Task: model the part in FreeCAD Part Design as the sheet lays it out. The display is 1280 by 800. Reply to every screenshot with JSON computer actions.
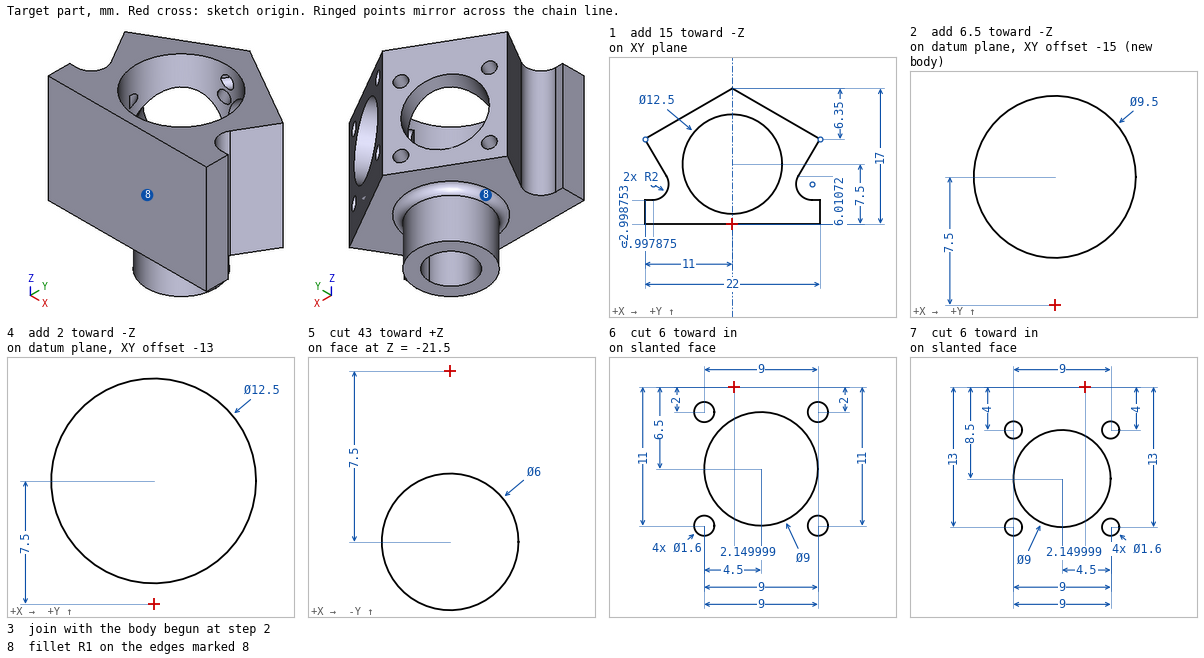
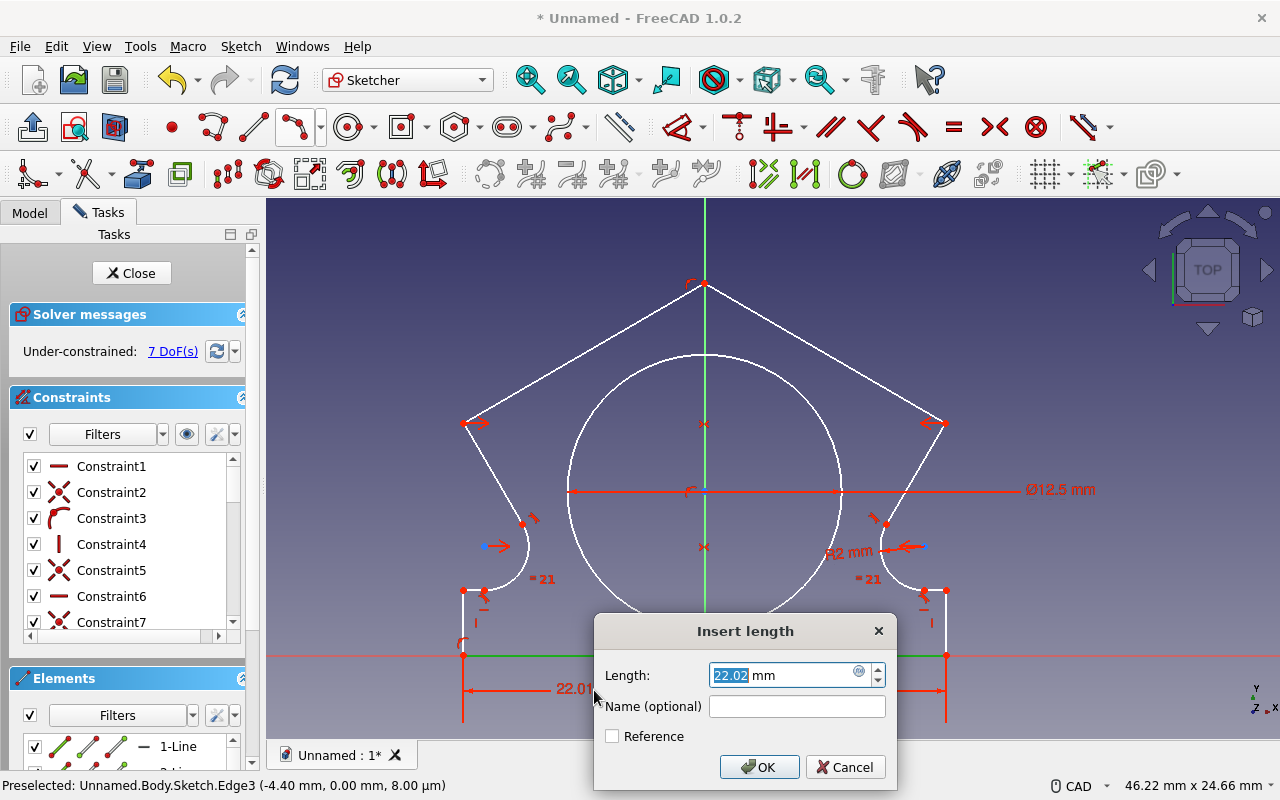
{"action": "type", "text": "22"}
{"action": "key", "text": "Return"}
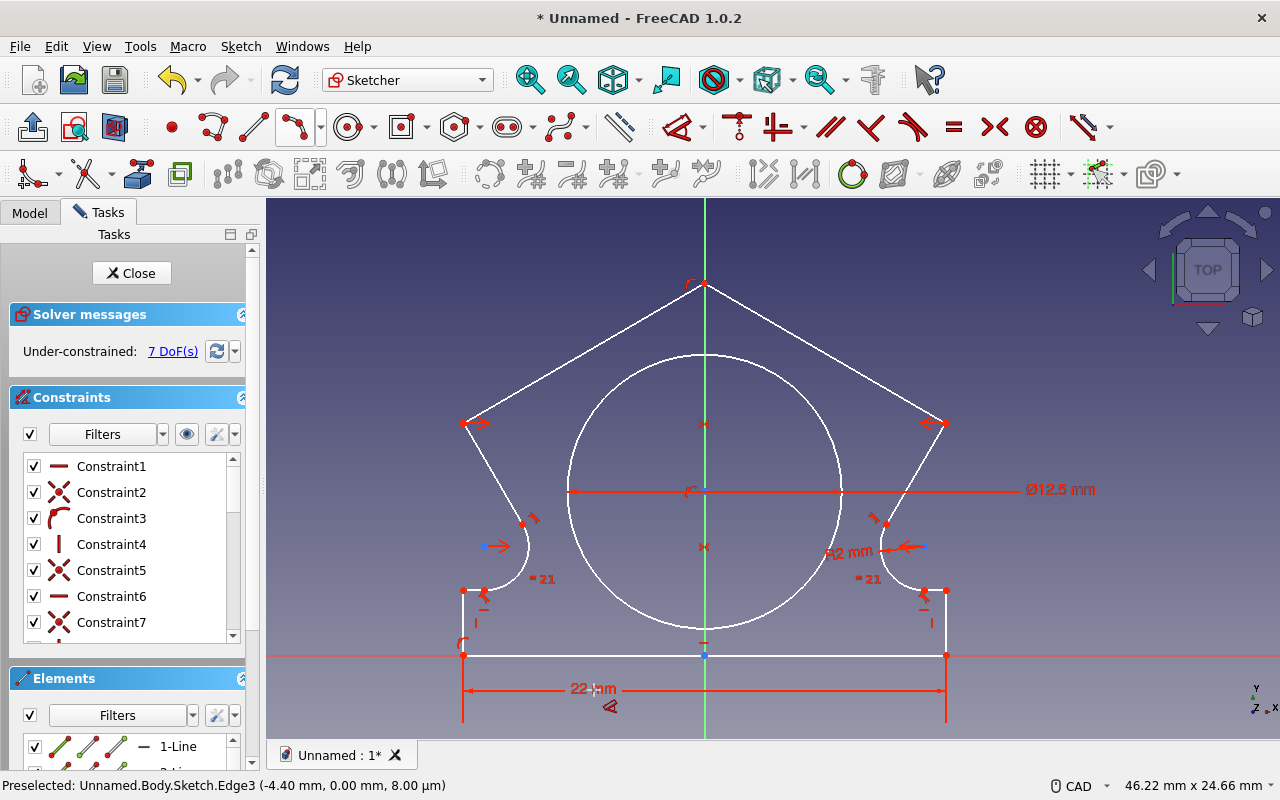
{"action": "left_click", "coordinate": [463, 590]}
{"action": "left_click", "coordinate": [500, 690]}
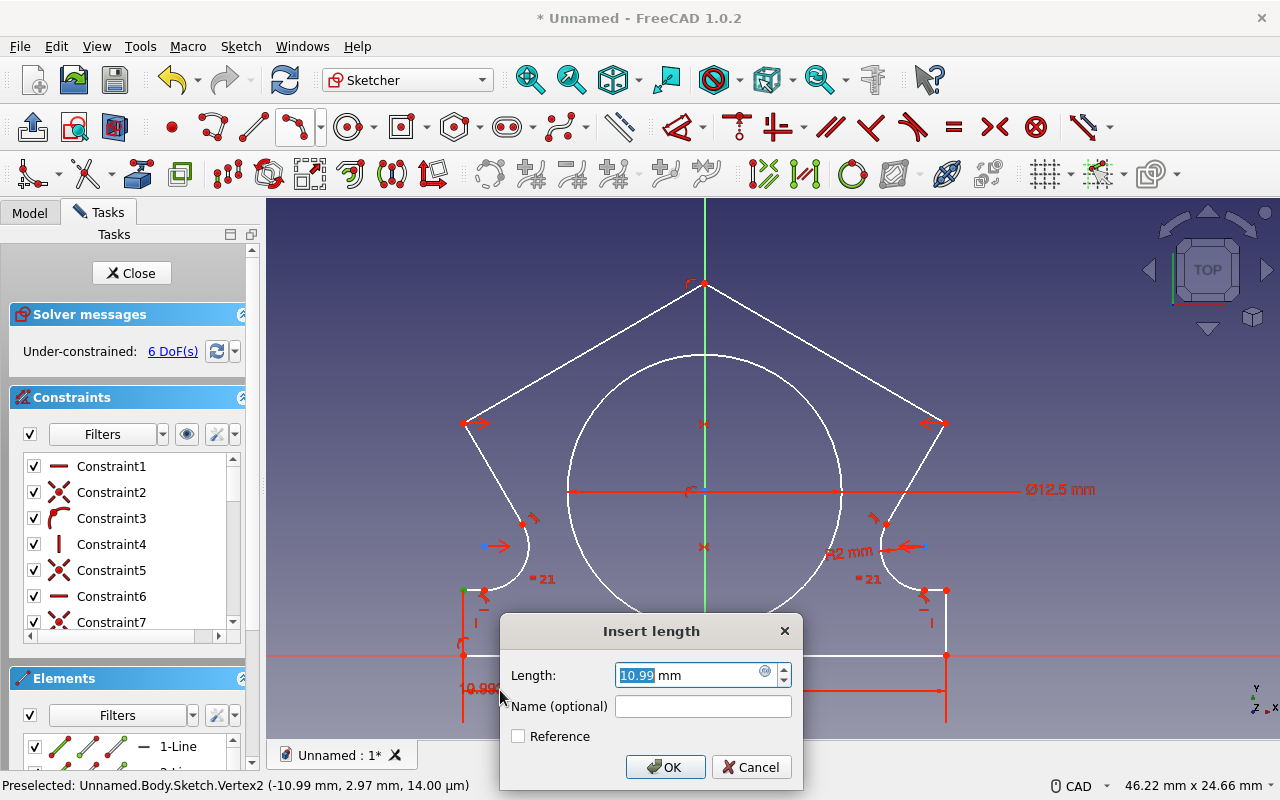
{"action": "type", "text": "11"}
{"action": "key", "text": "Return"}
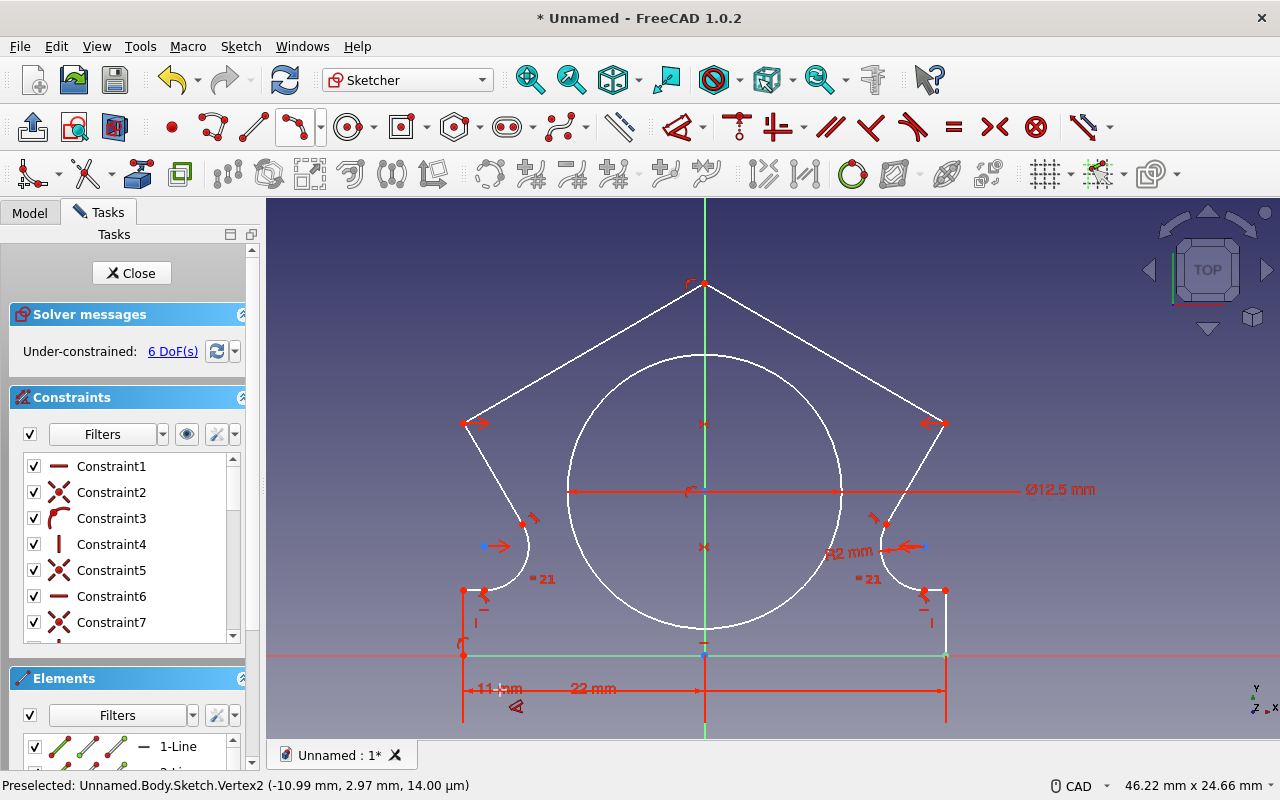
{"action": "left_click", "coordinate": [705, 283]}
{"action": "left_click", "coordinate": [739, 469]}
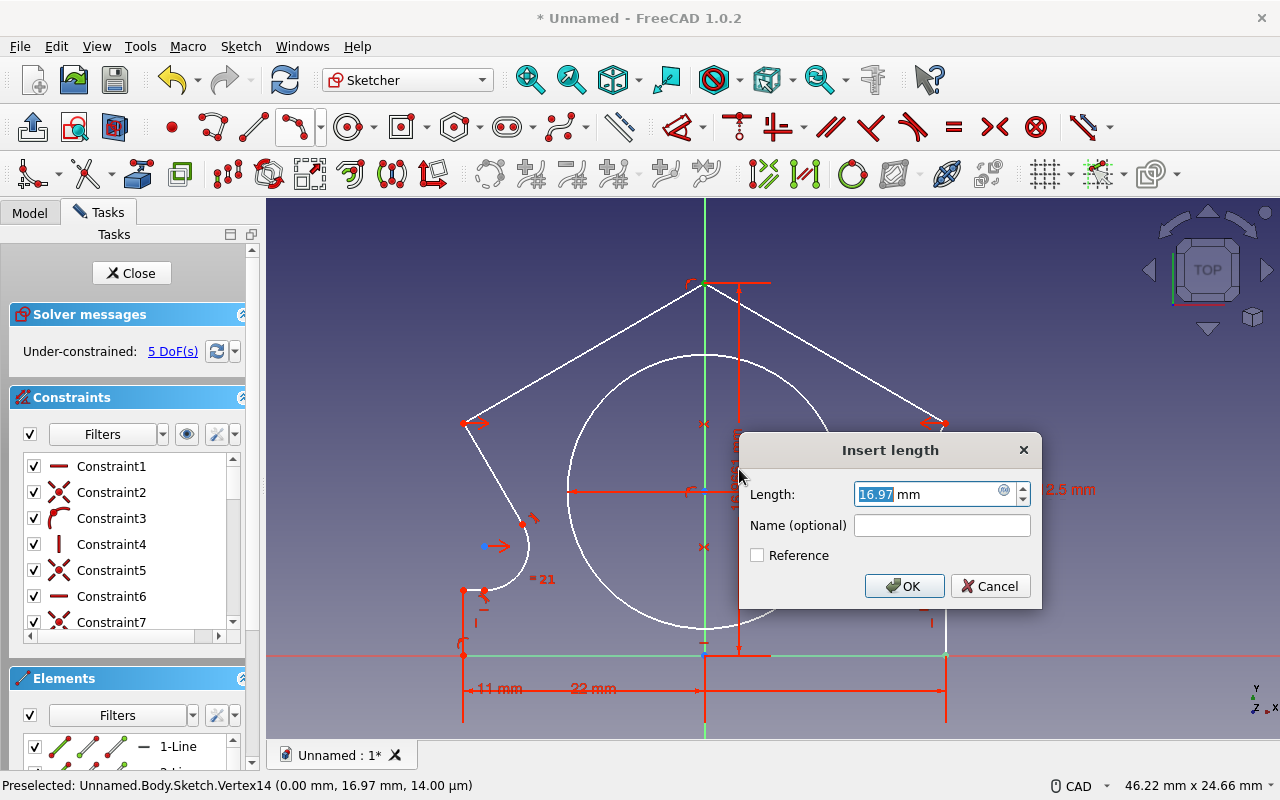
{"action": "type", "text": "17"}
{"action": "key", "text": "Return"}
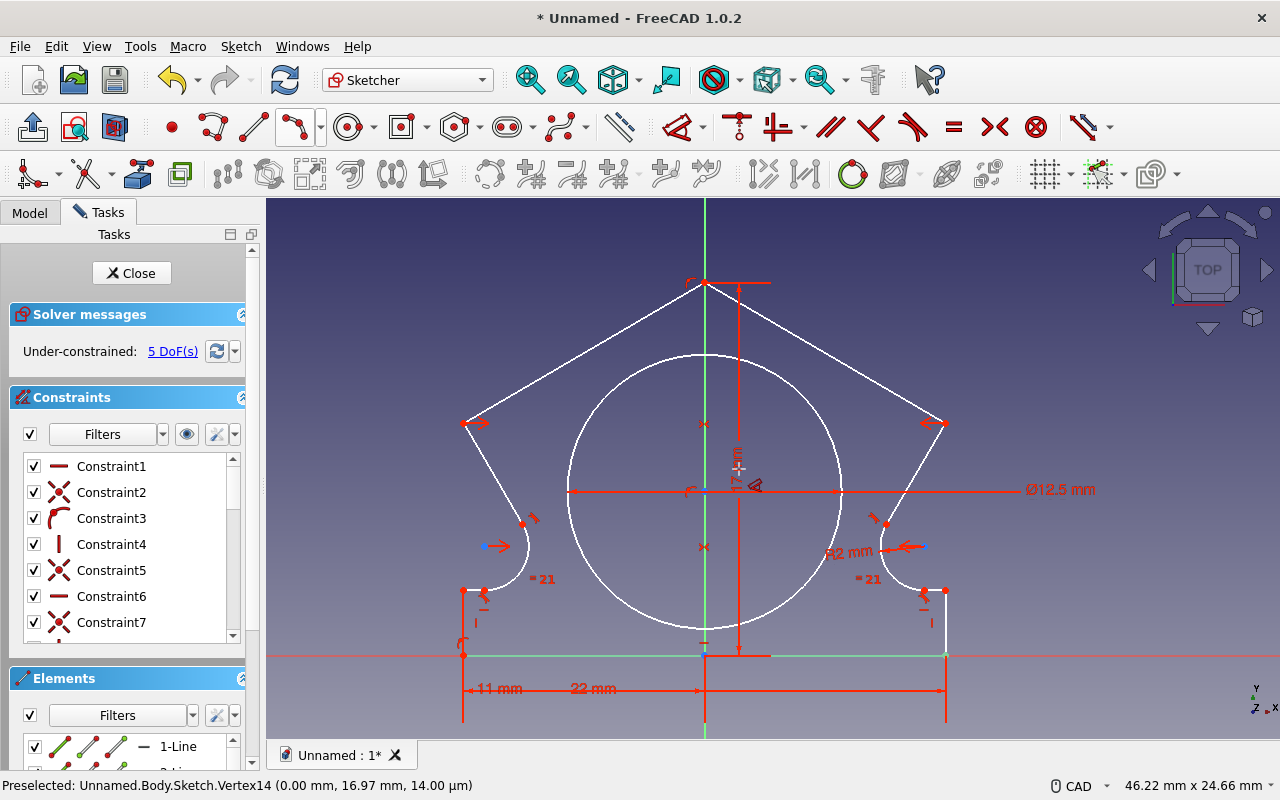
{"action": "left_click", "coordinate": [705, 492]}
{"action": "left_click", "coordinate": [739, 574]}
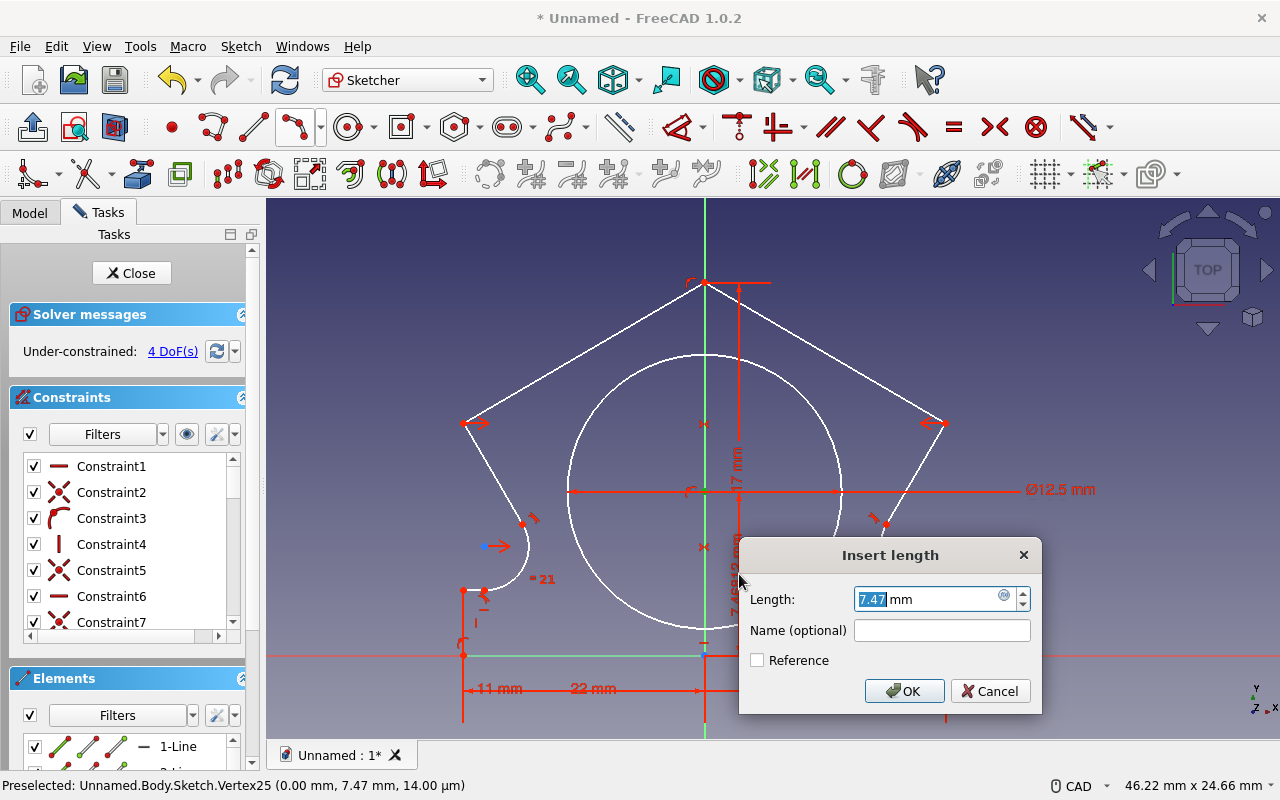
{"action": "type", "text": "7.5"}
{"action": "key", "text": "Return"}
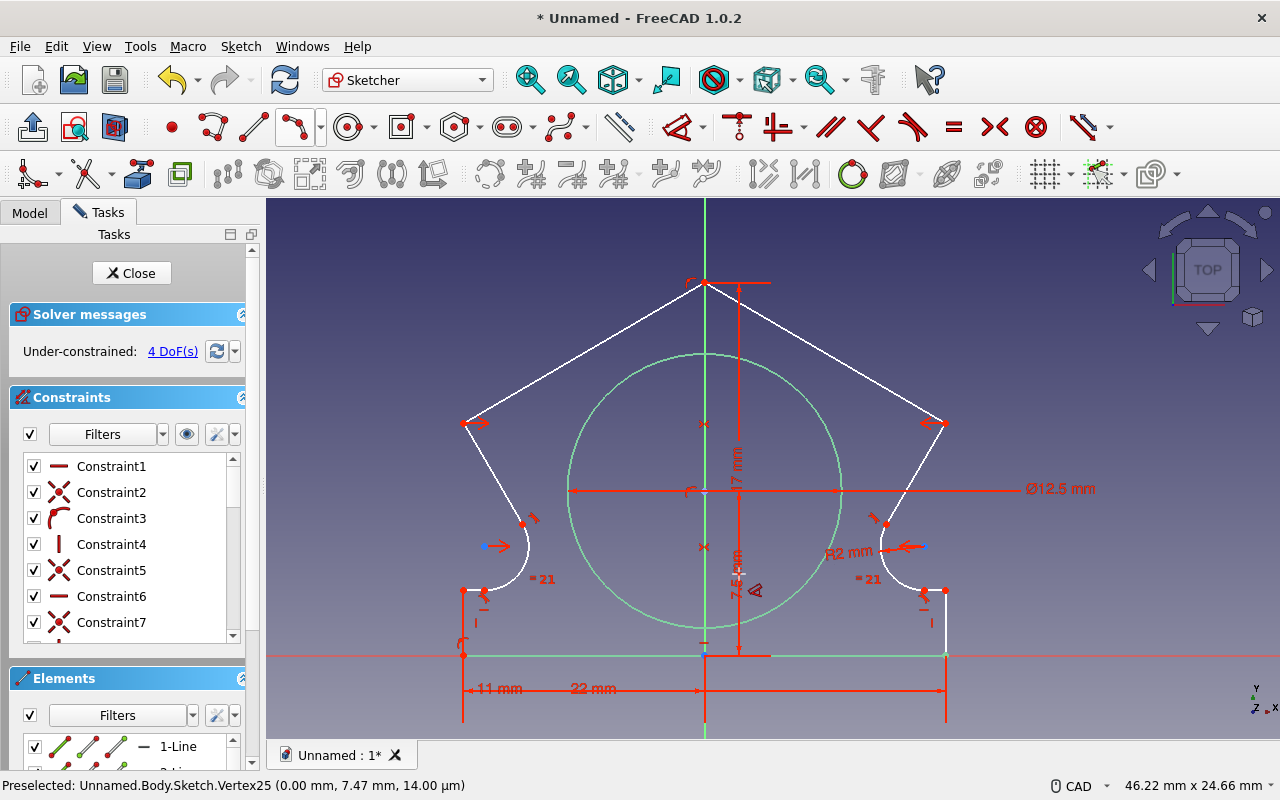
{"action": "left_click", "coordinate": [873, 381]}
{"action": "left_click", "coordinate": [979, 353]}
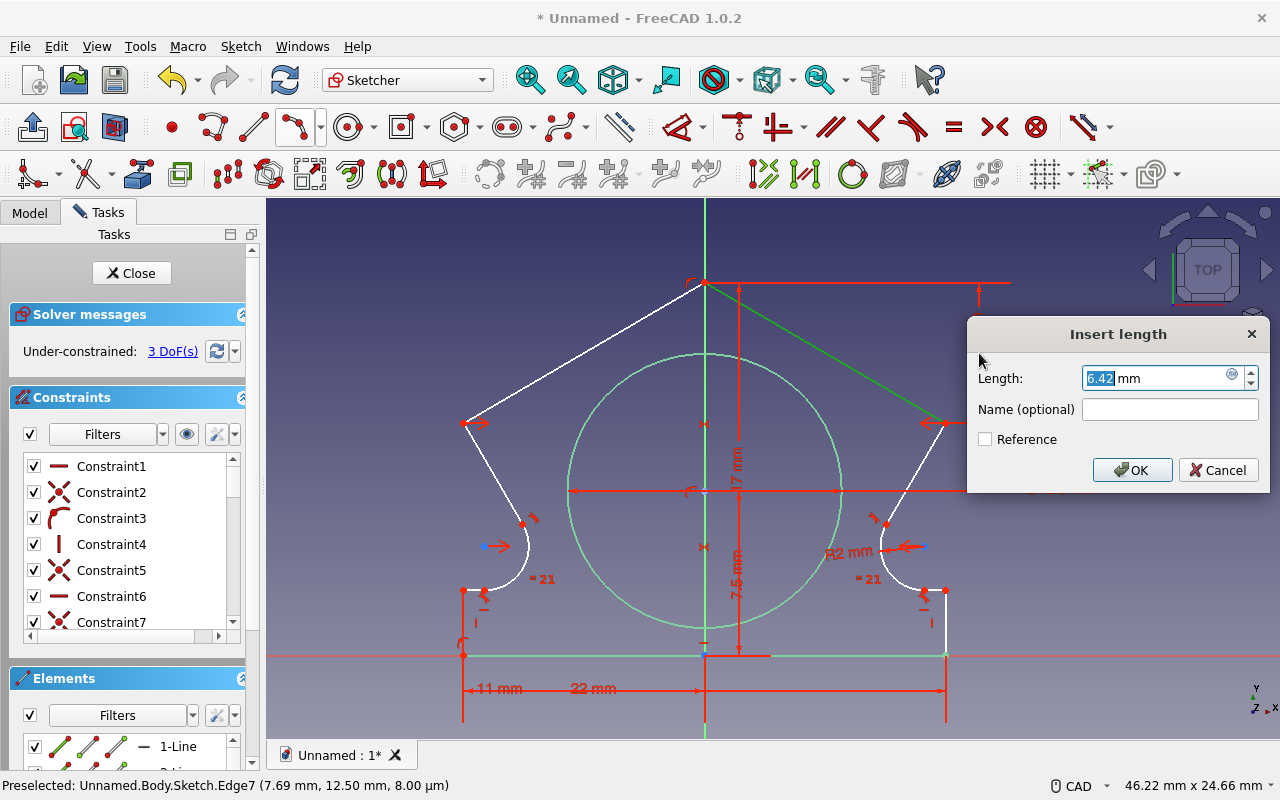
{"action": "type", "text": "6.35"}
{"action": "key", "text": "Return"}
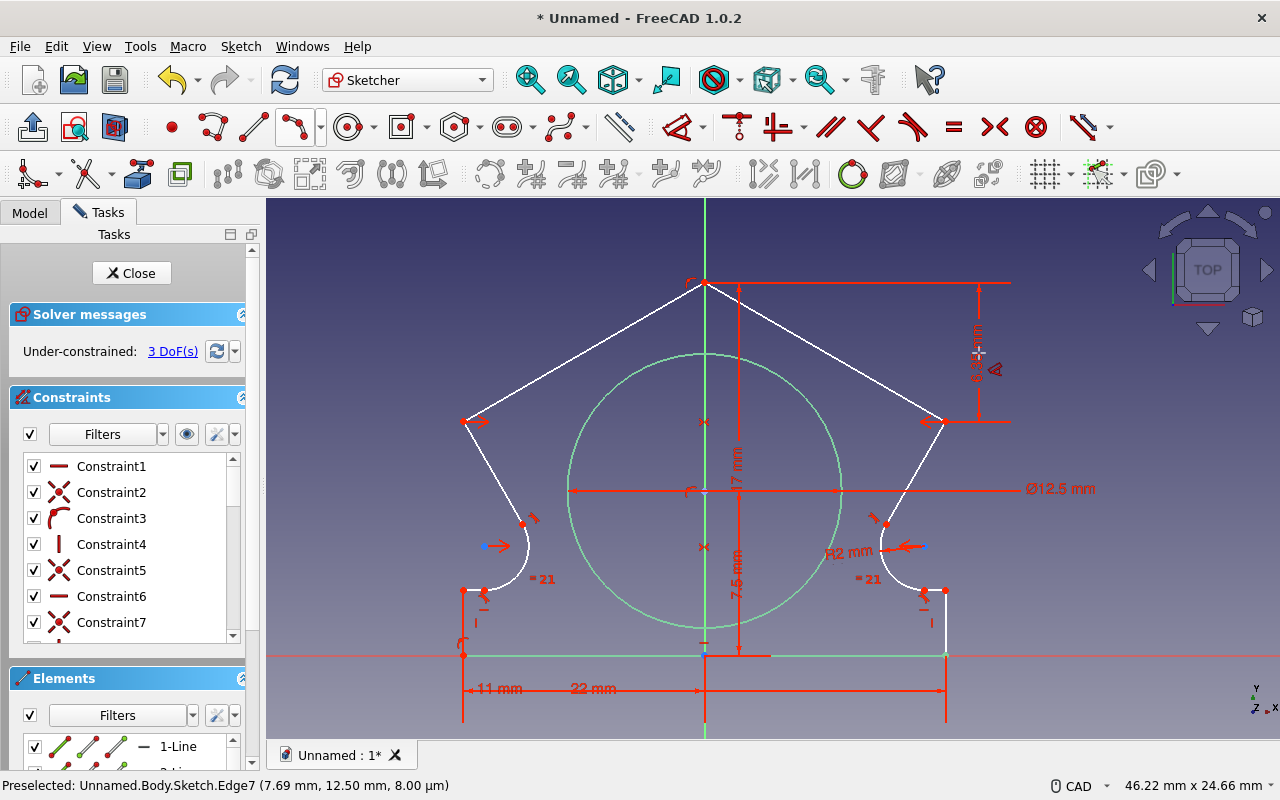
{"action": "scroll", "coordinate": [474, 590], "scroll_direction": "up", "scroll_amount": 3}